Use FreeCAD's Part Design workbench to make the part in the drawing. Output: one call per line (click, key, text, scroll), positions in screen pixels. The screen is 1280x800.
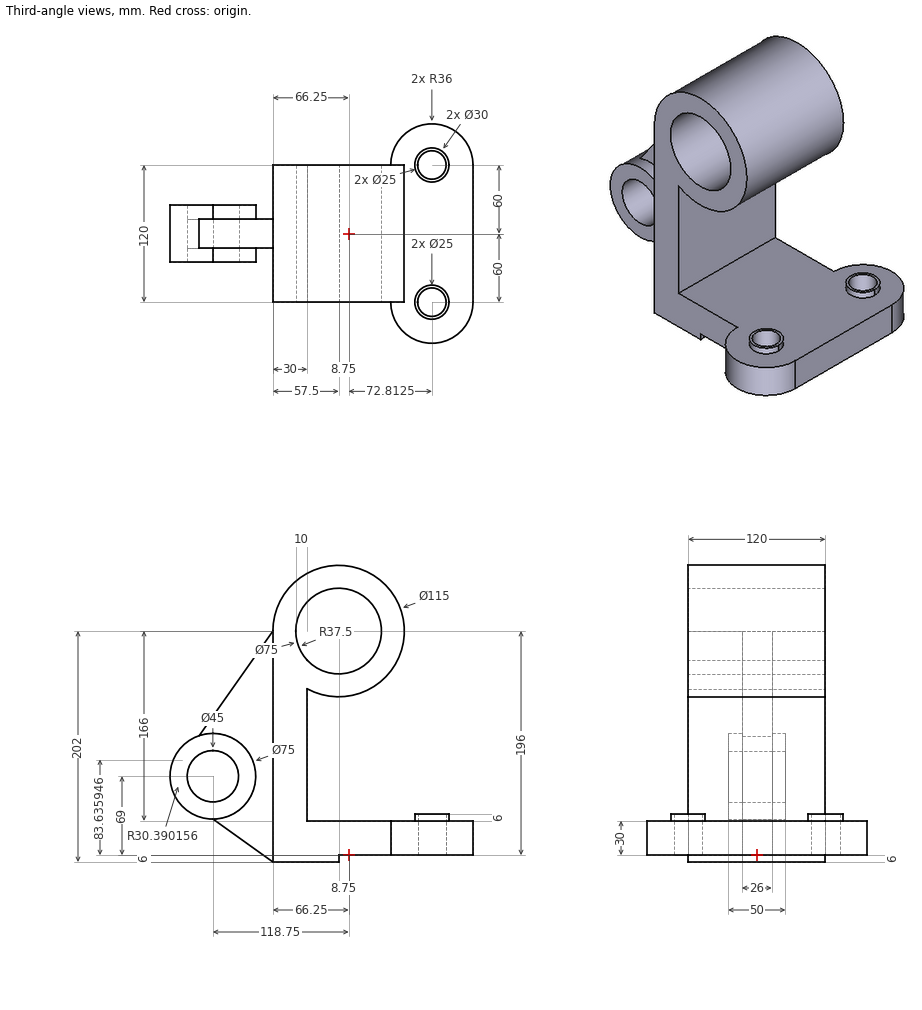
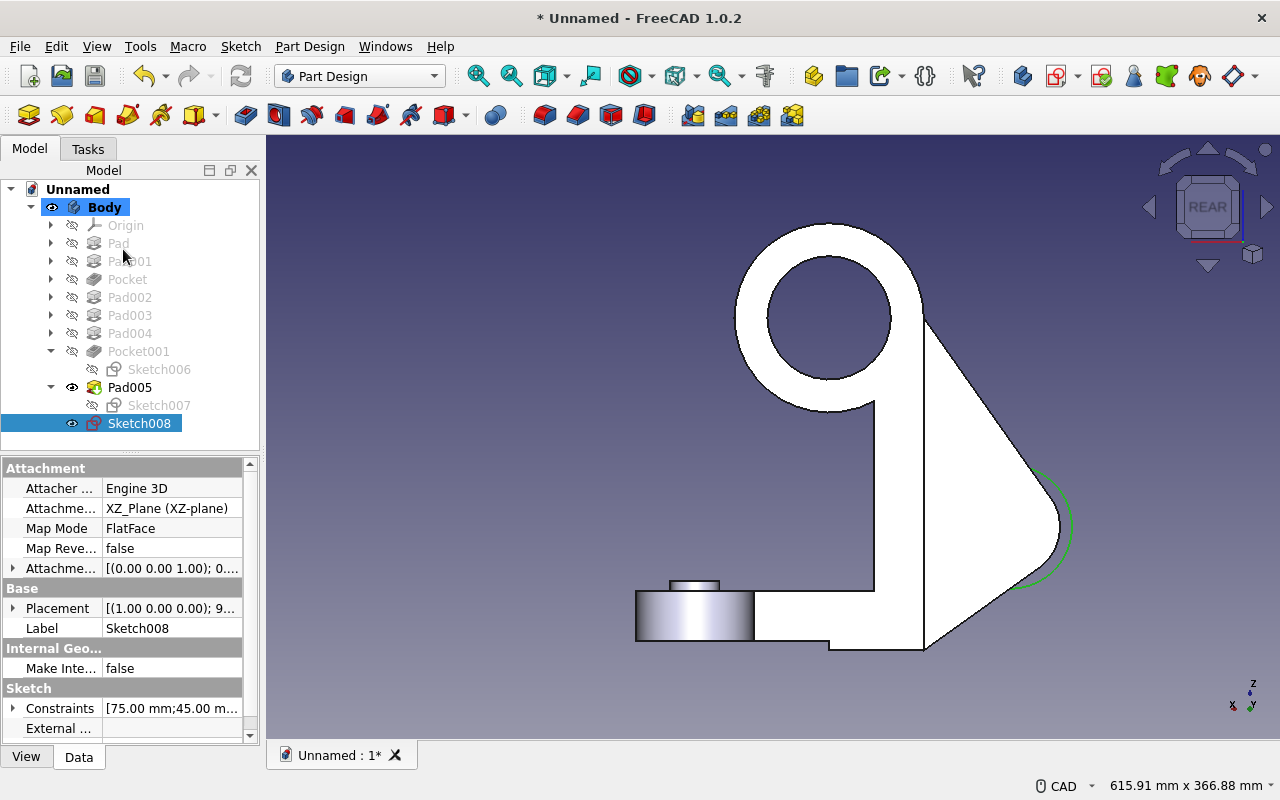
click(29, 116)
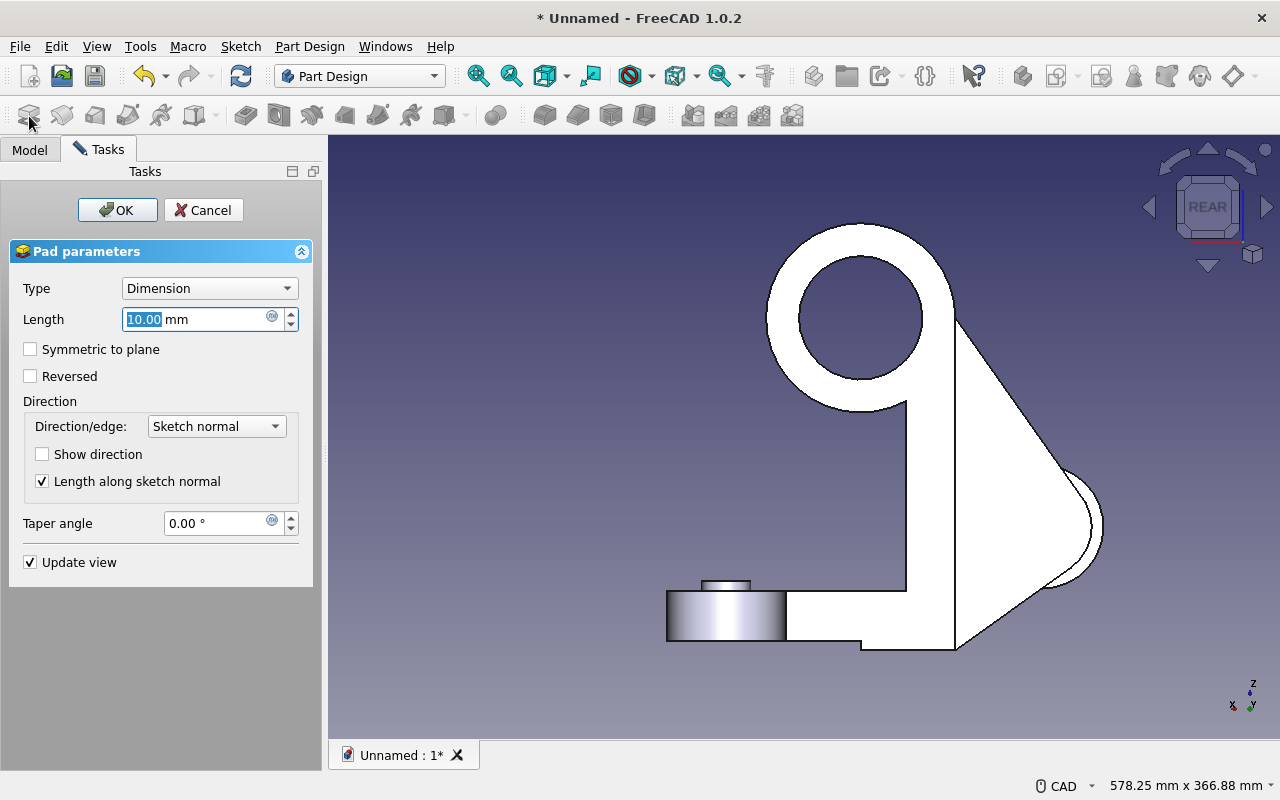
text(50)
key(Tab)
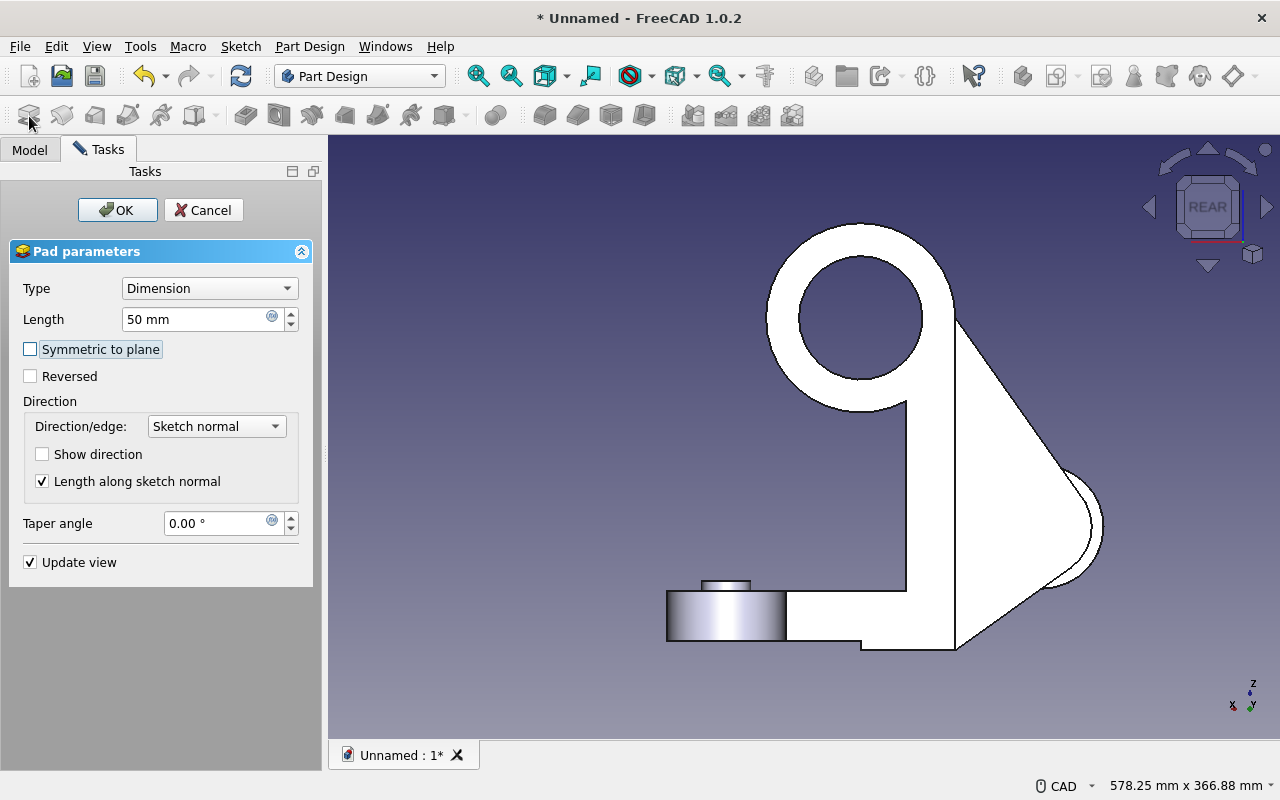
click(31, 349)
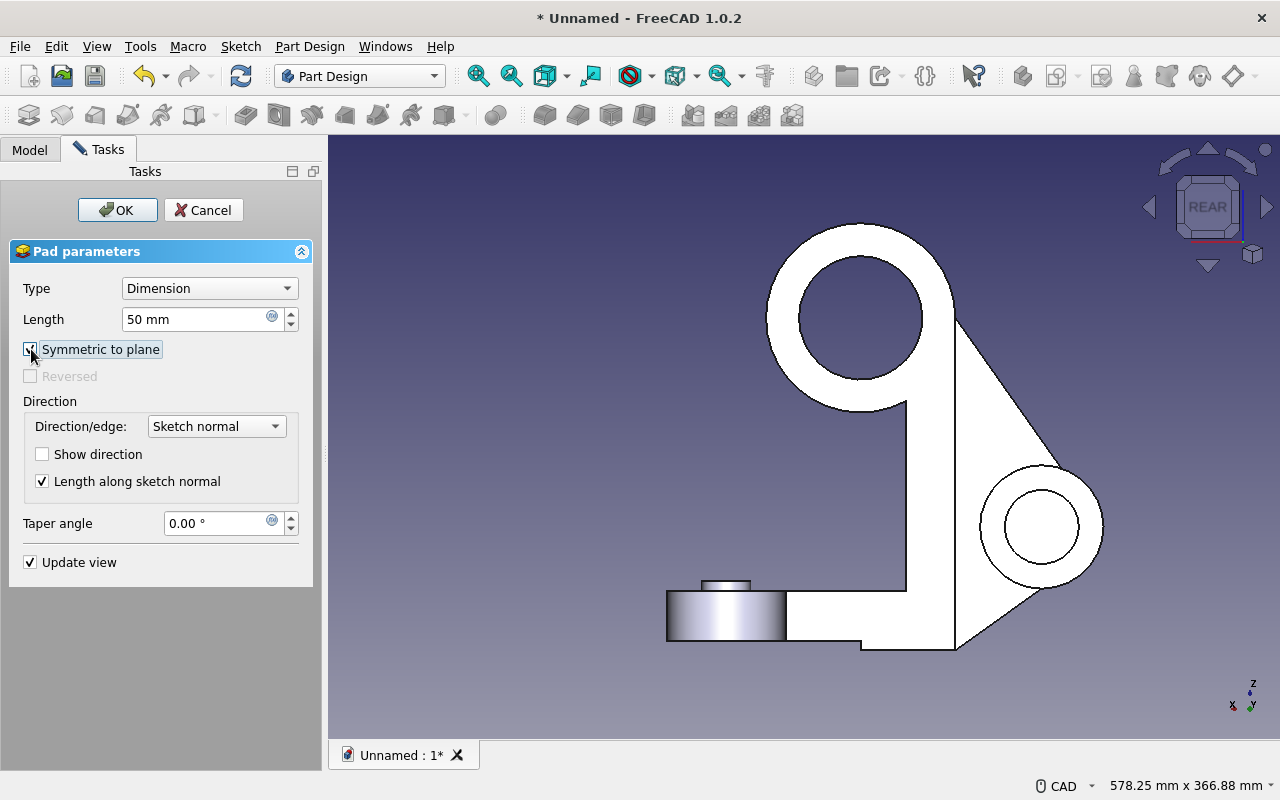
click(118, 210)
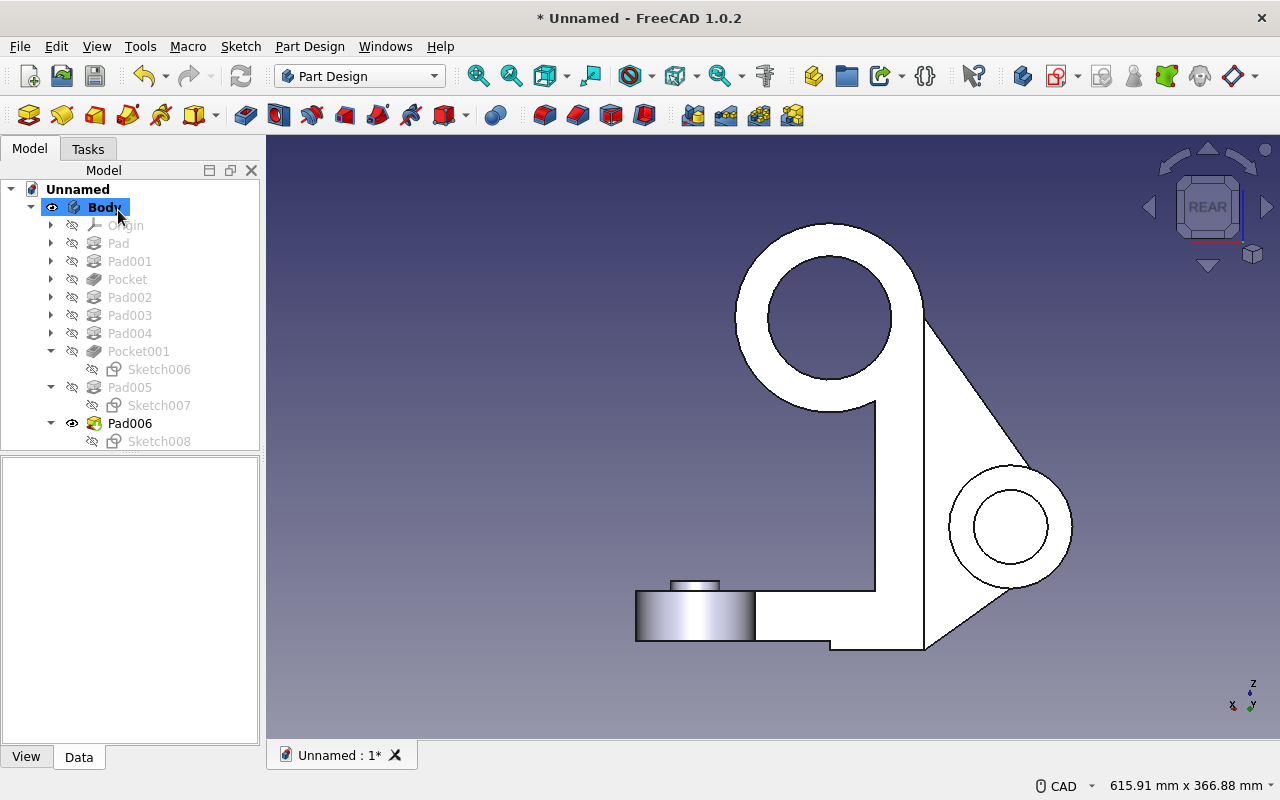
click(962, 436)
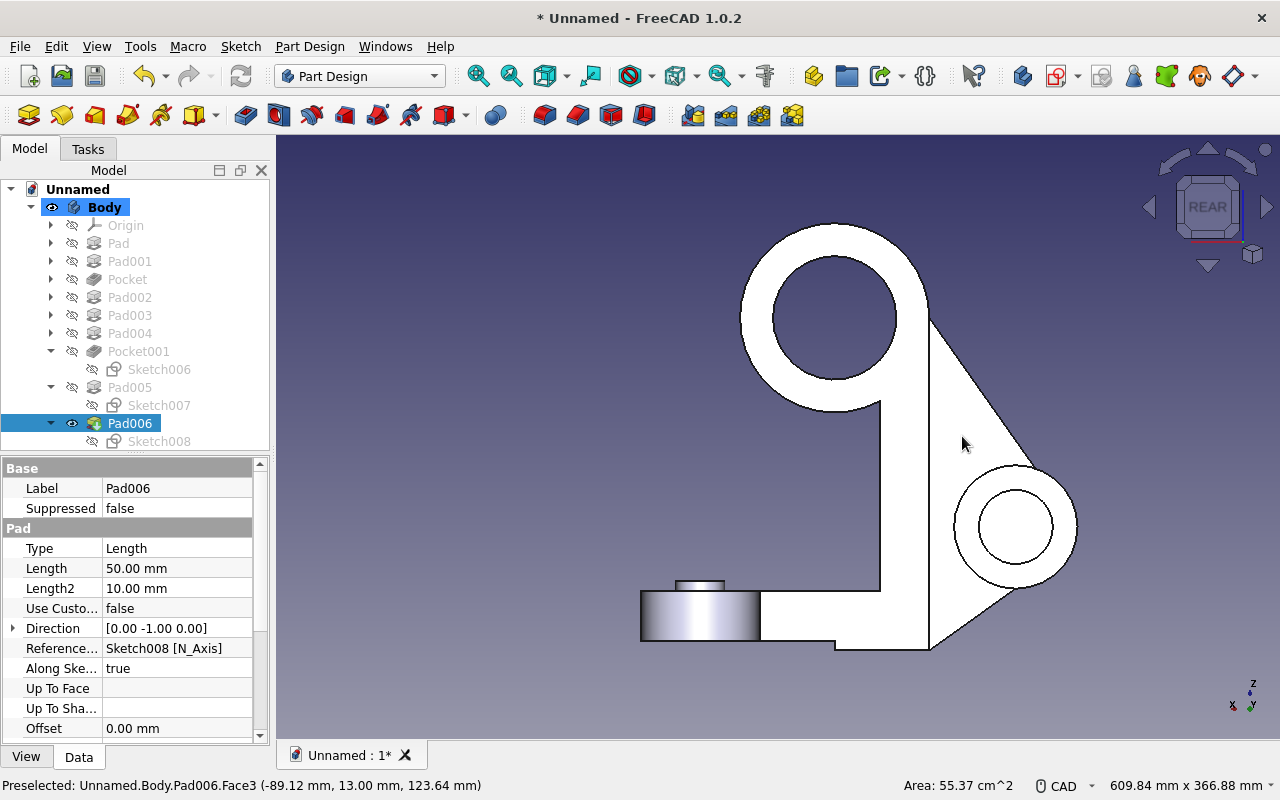
click(1056, 76)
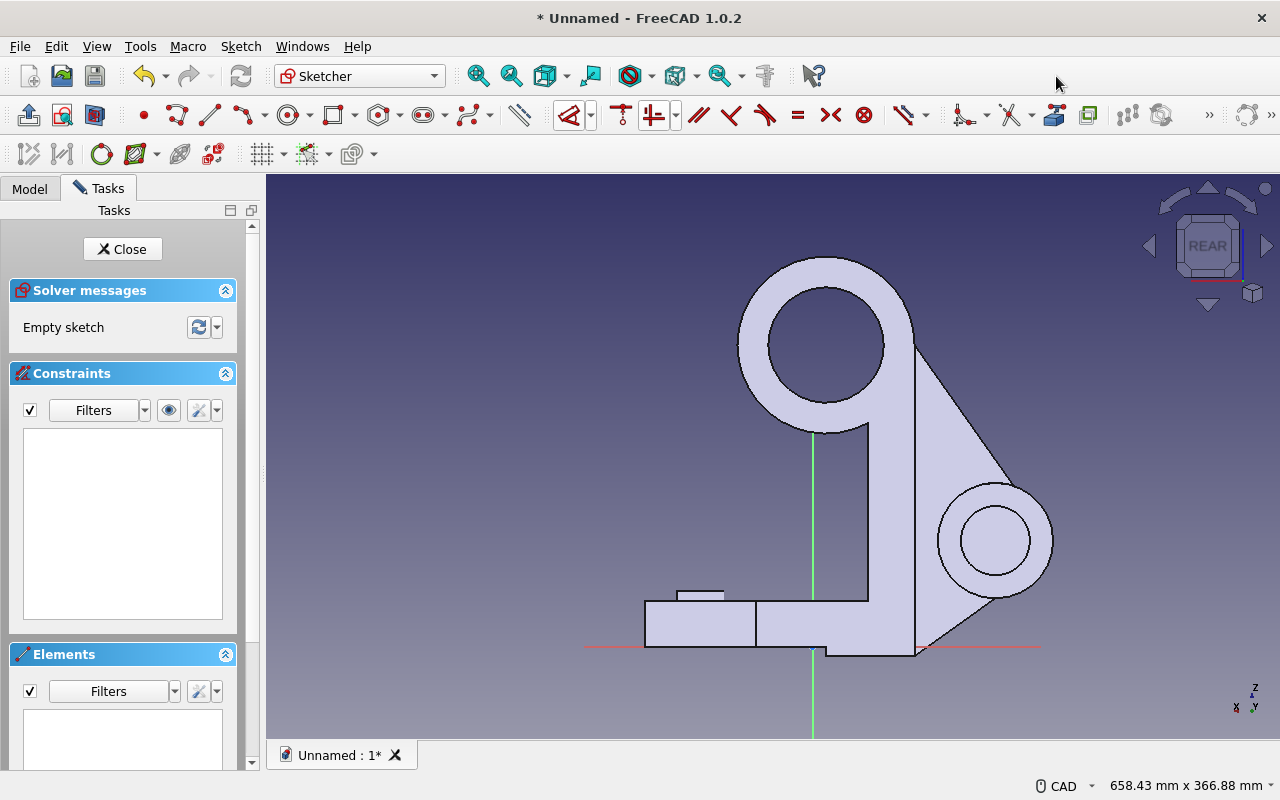
scroll(1069, 562, up, 8)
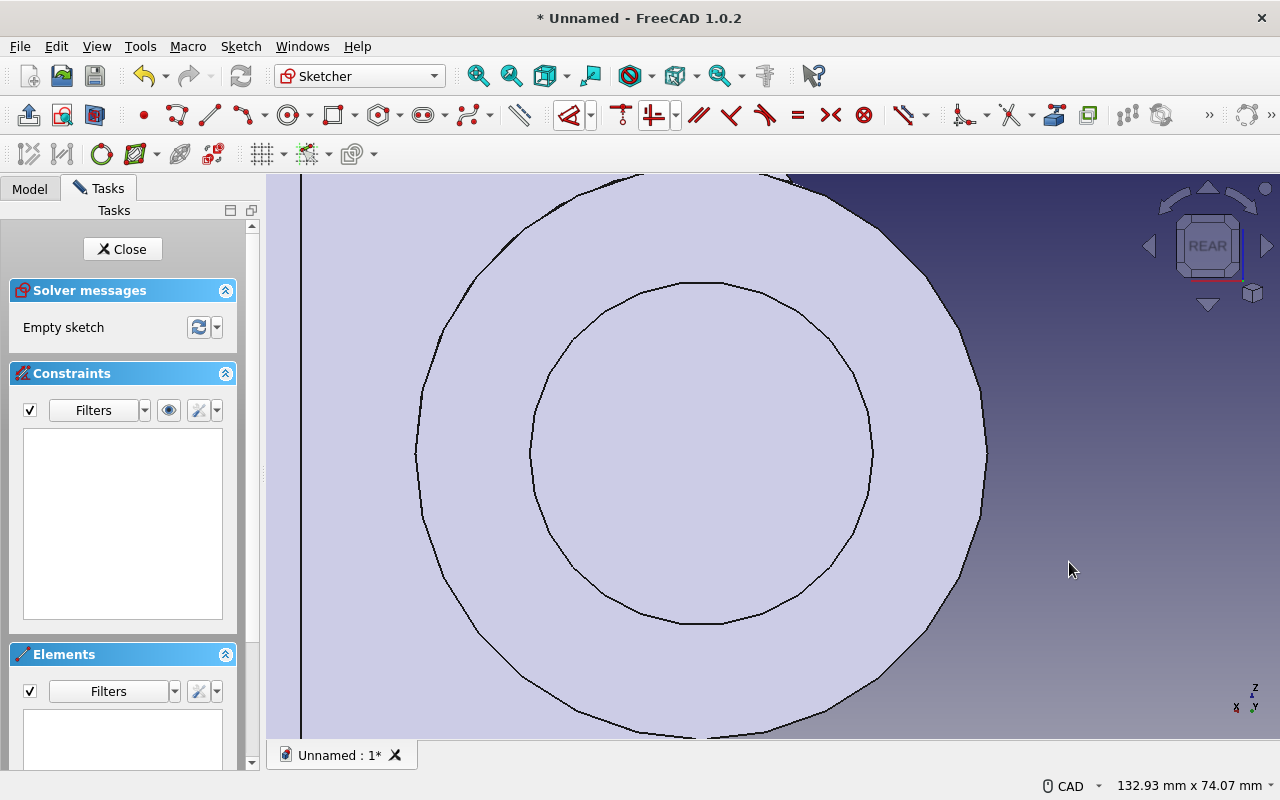
click(288, 116)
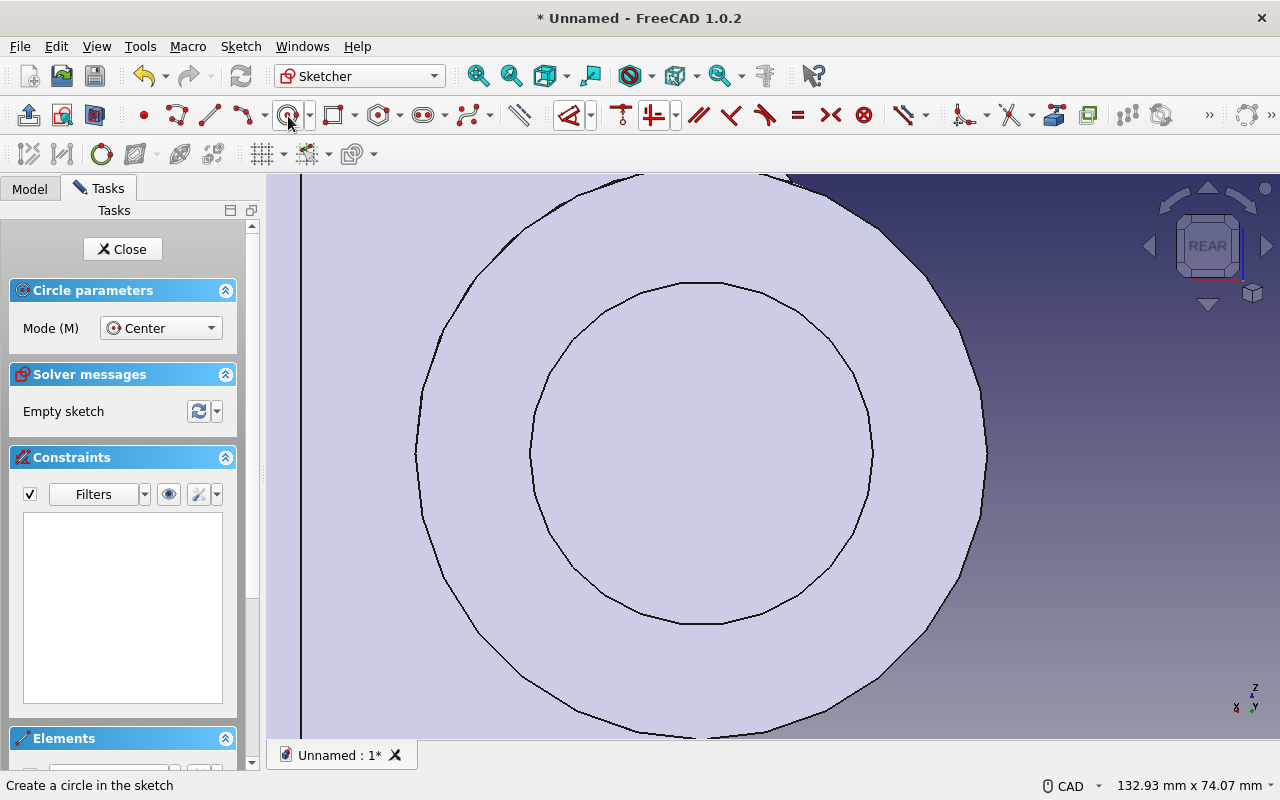
click(701, 454)
click(823, 332)
key(Escape)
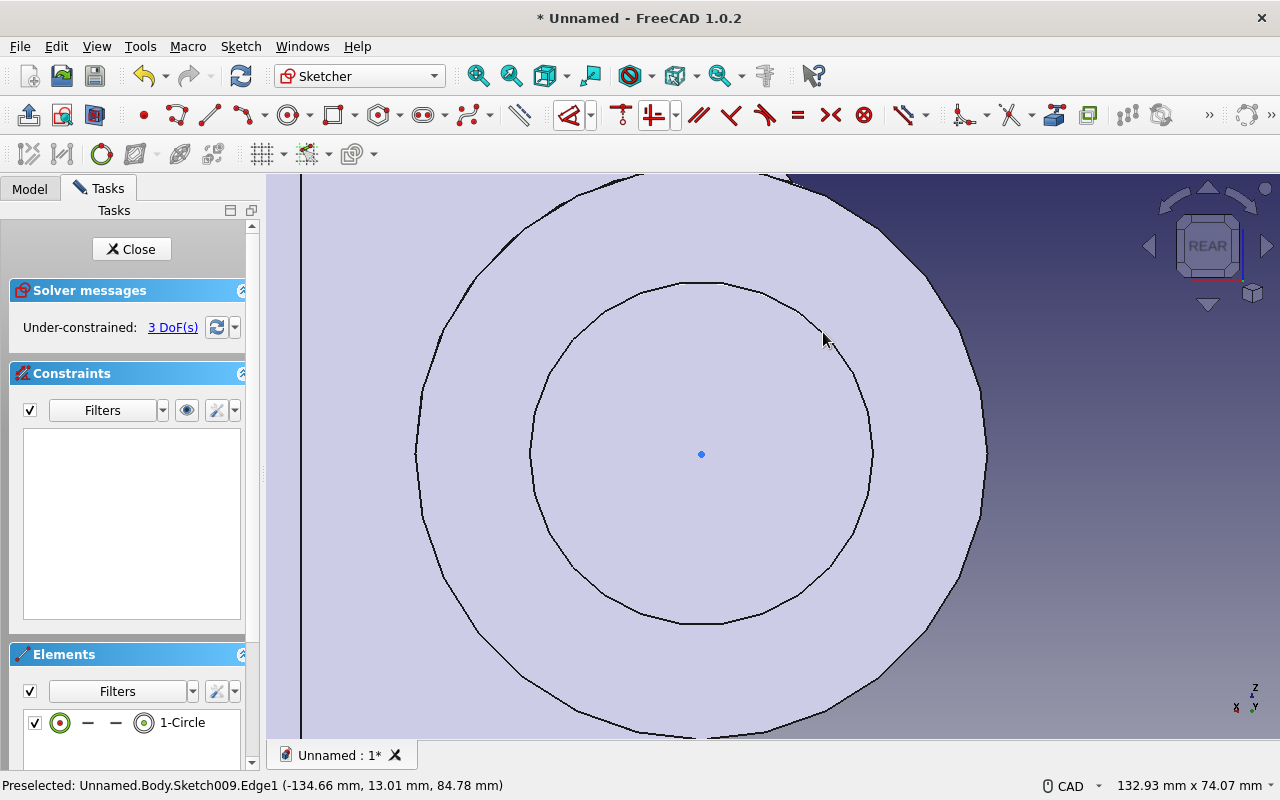
click(823, 333)